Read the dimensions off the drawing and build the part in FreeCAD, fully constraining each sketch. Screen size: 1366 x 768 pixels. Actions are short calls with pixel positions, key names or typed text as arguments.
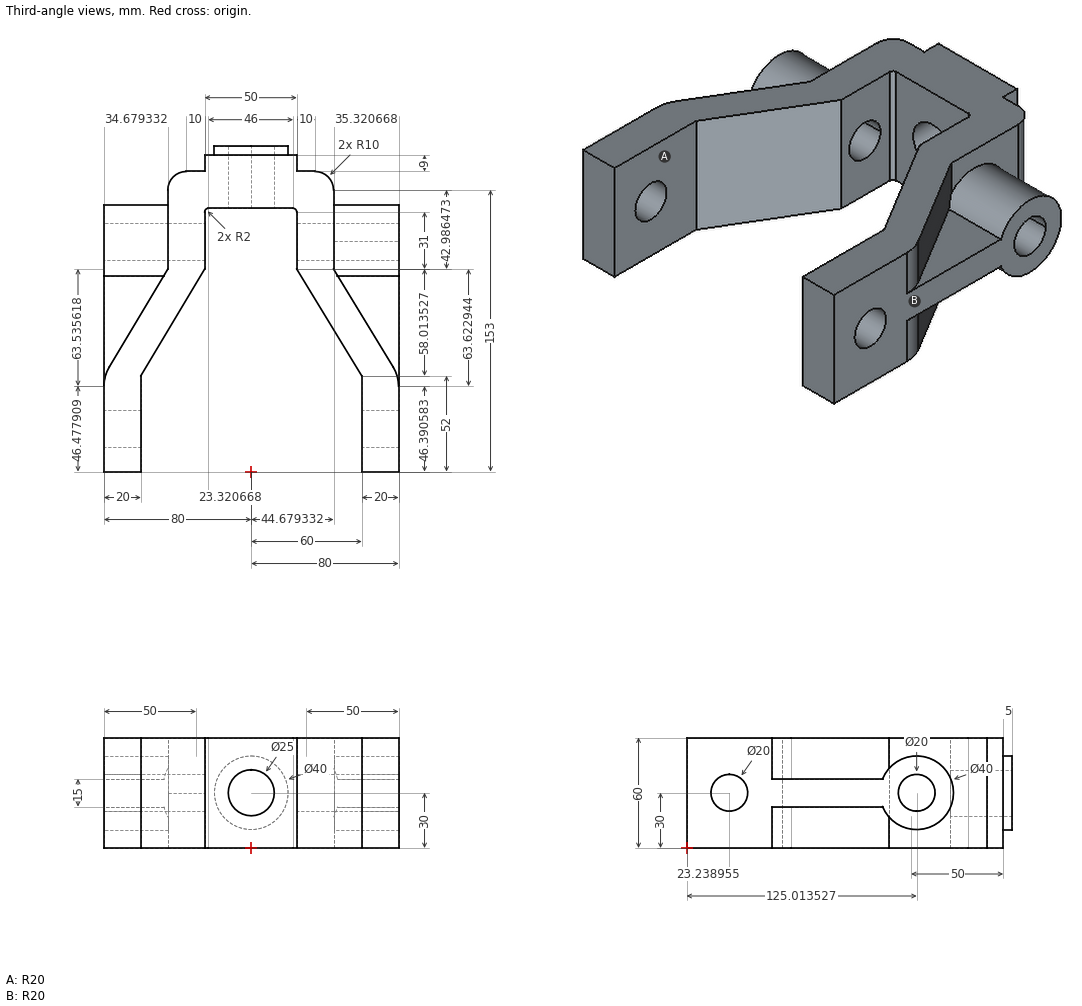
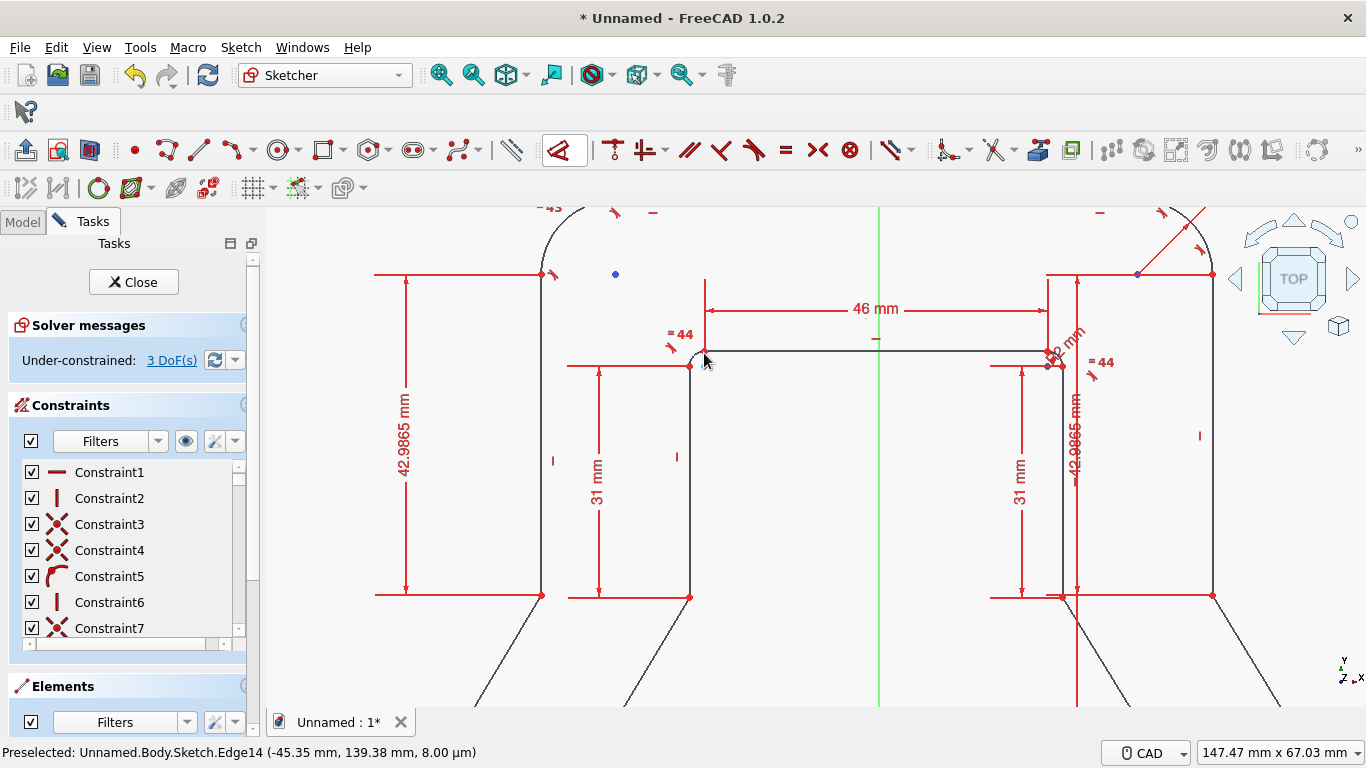
click(705, 351)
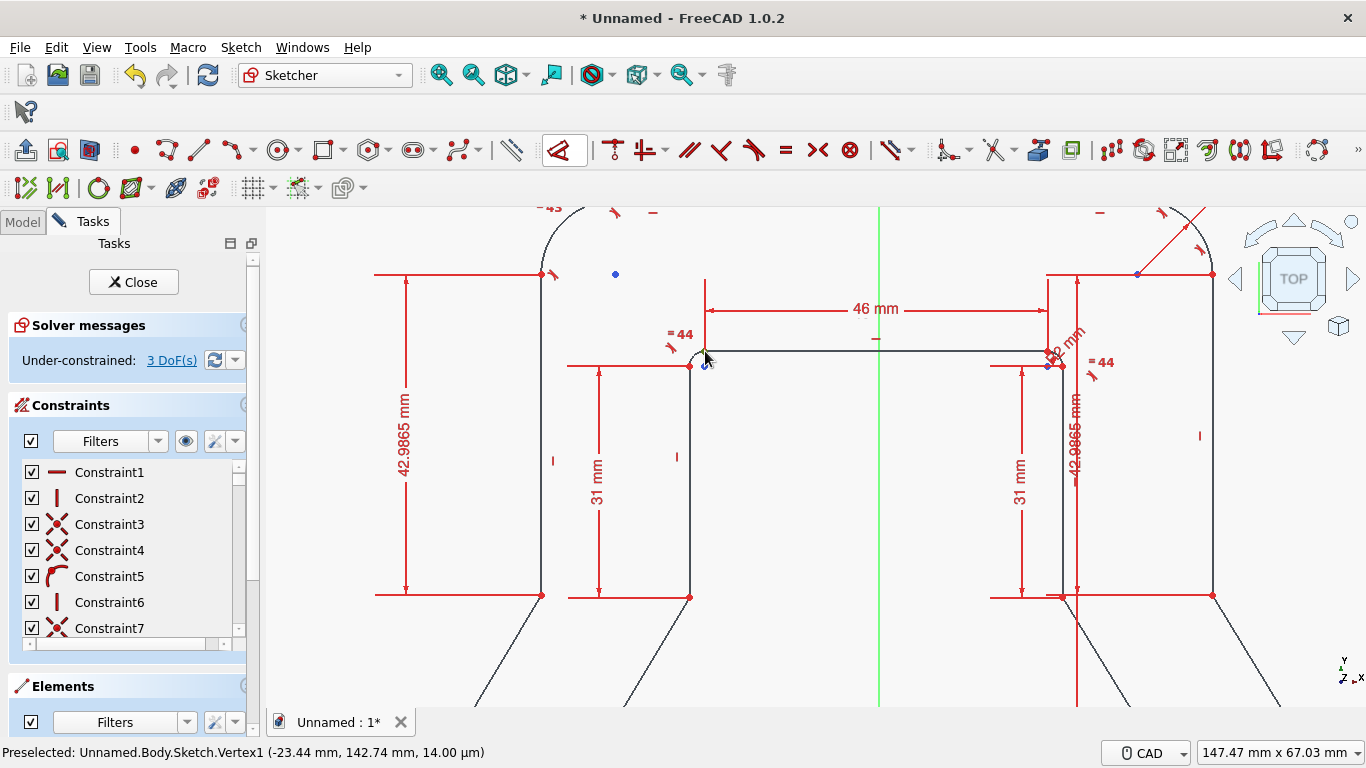
key(l)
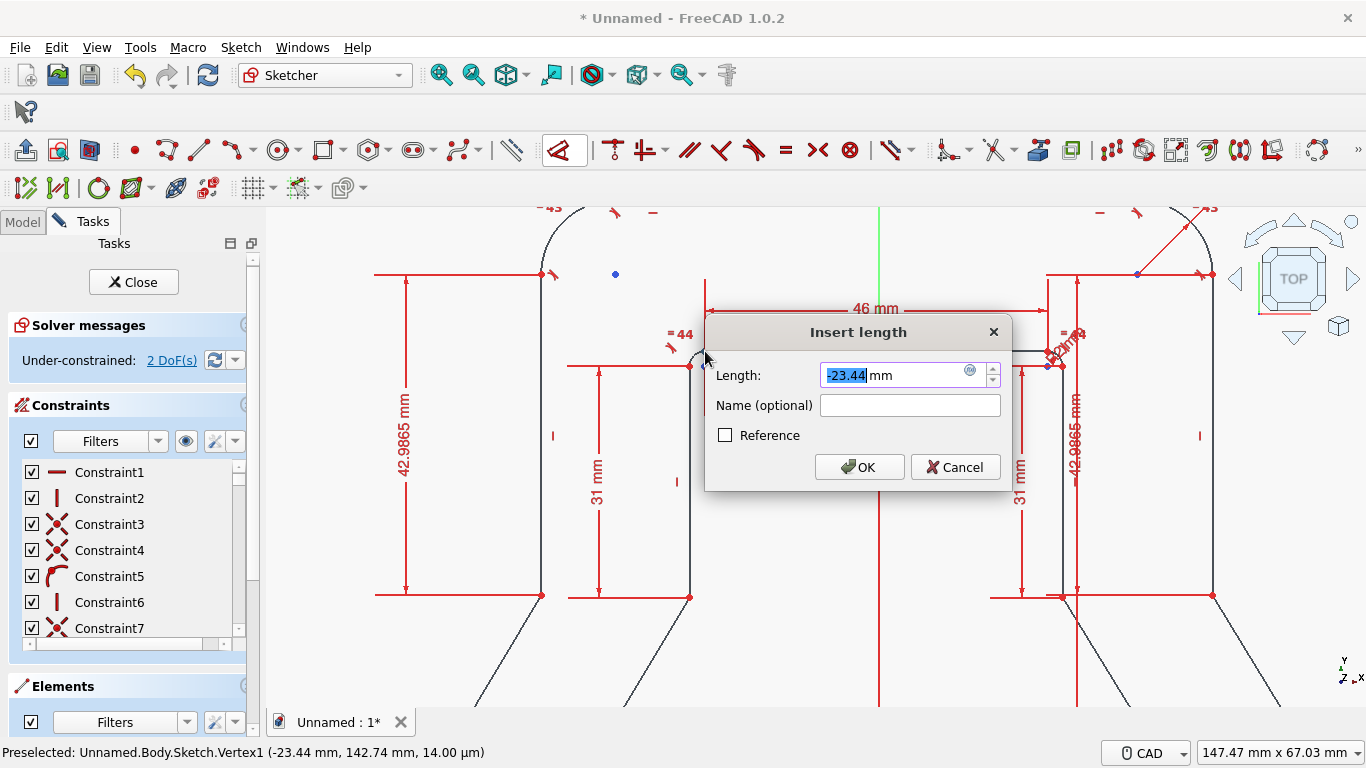
text(-23.320668)
key(Return)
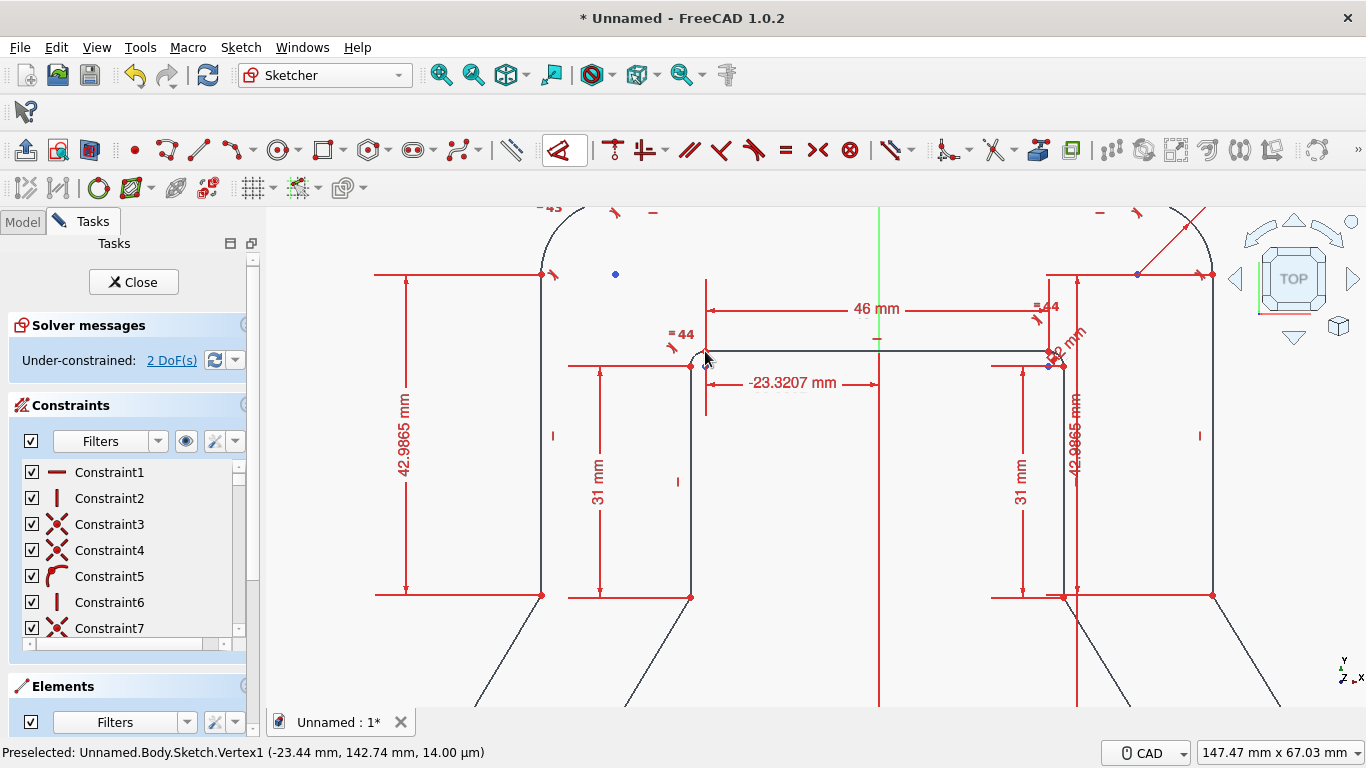
scroll(704, 353, down, 7)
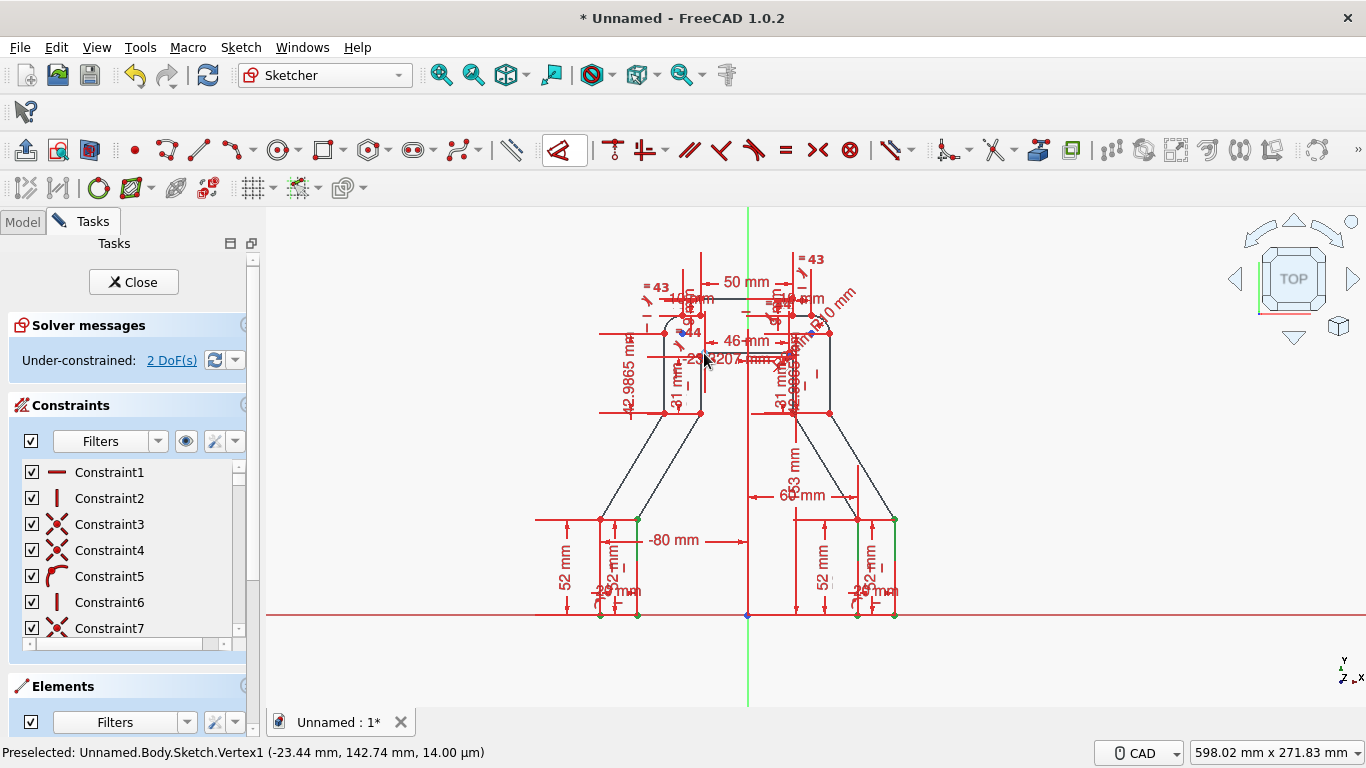
click(830, 413)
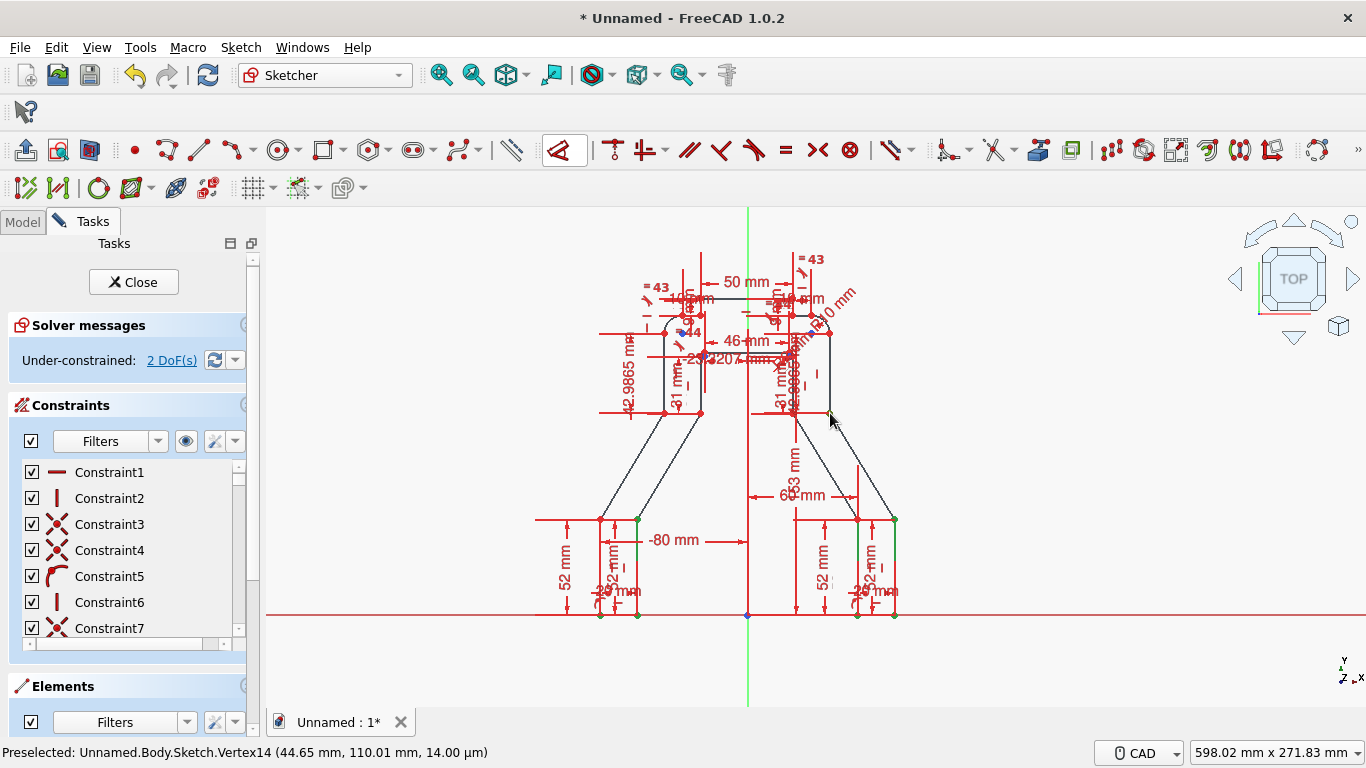
key(l)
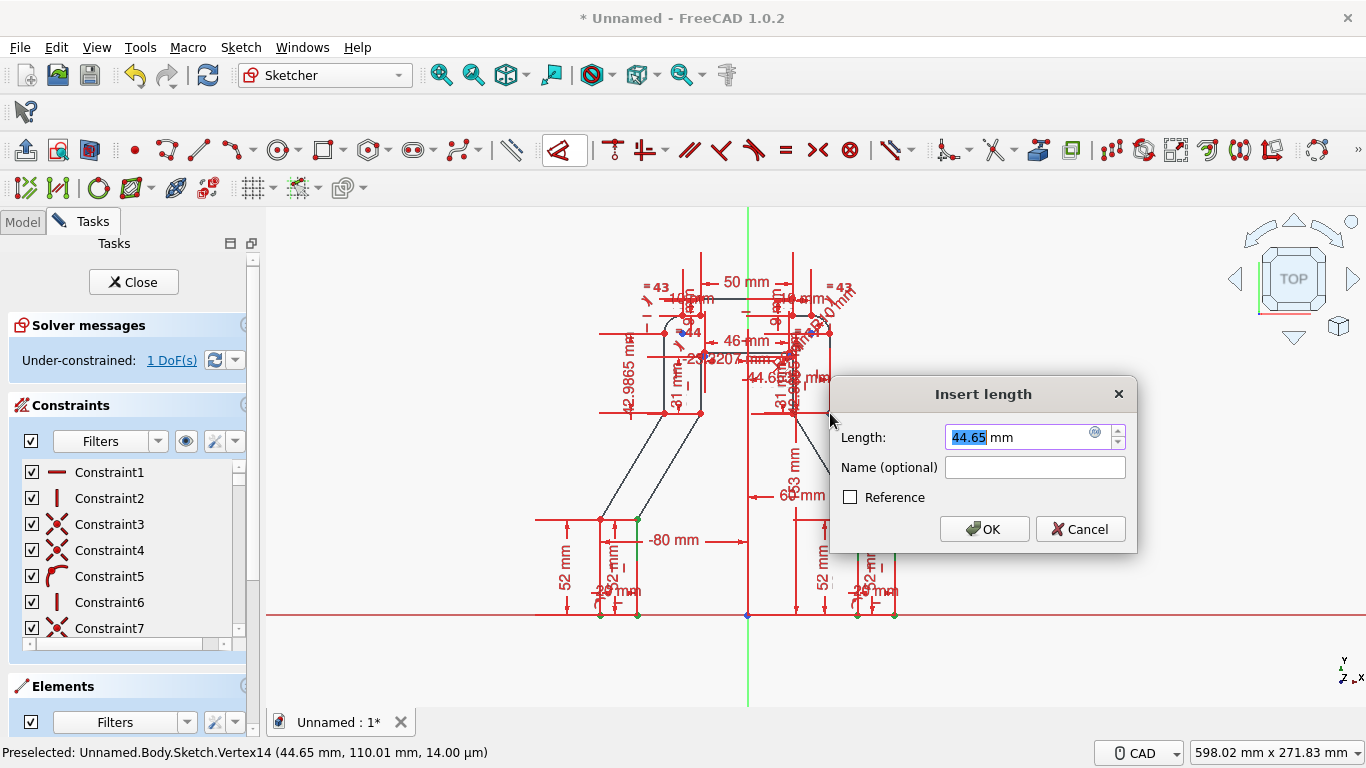
text(44.679332)
key(Return)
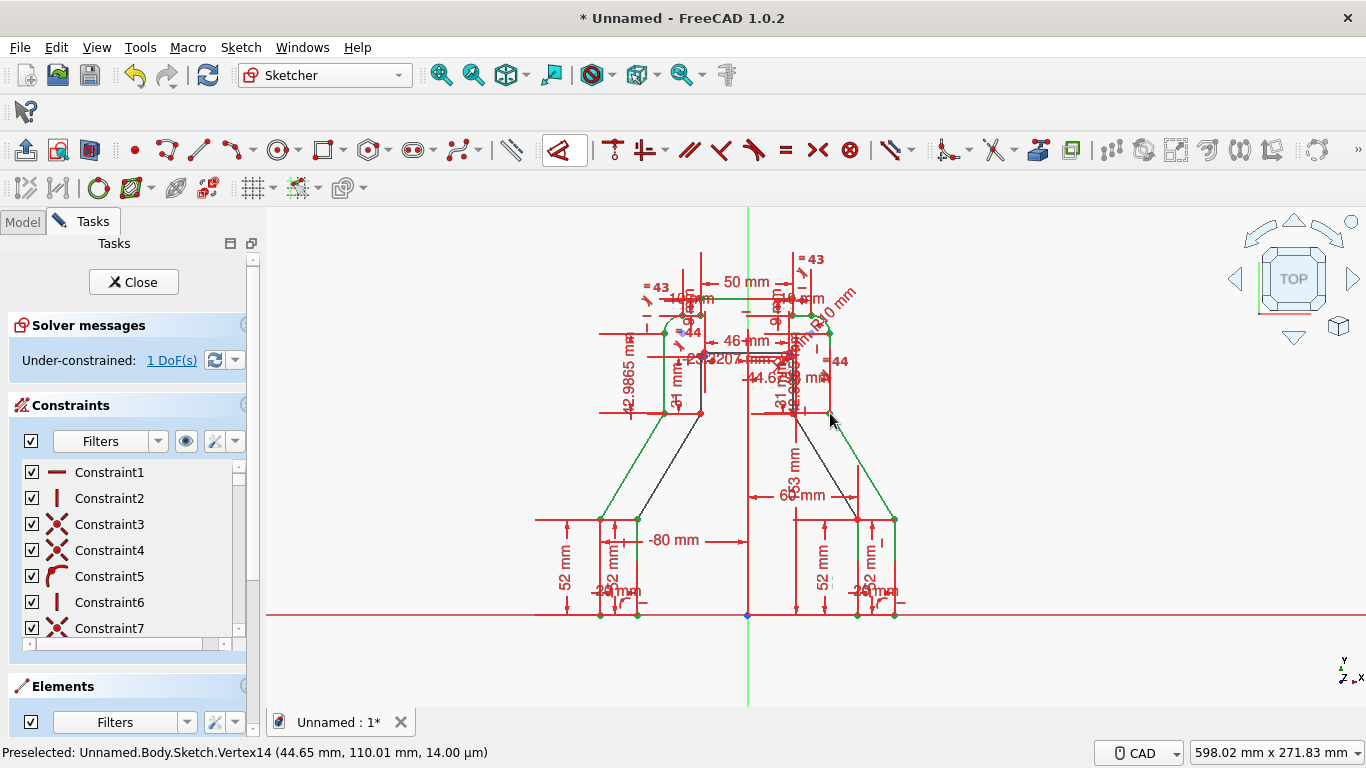
click(812, 445)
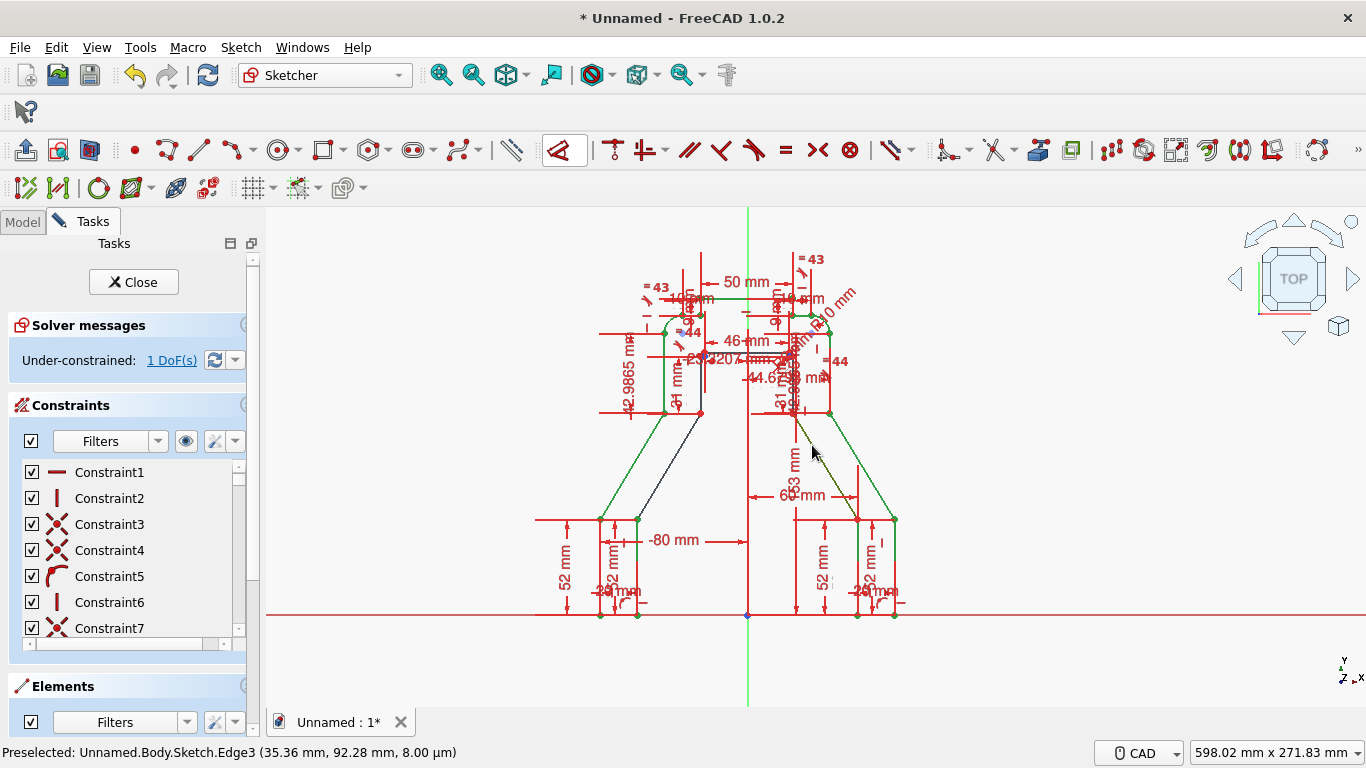
click(582, 150)